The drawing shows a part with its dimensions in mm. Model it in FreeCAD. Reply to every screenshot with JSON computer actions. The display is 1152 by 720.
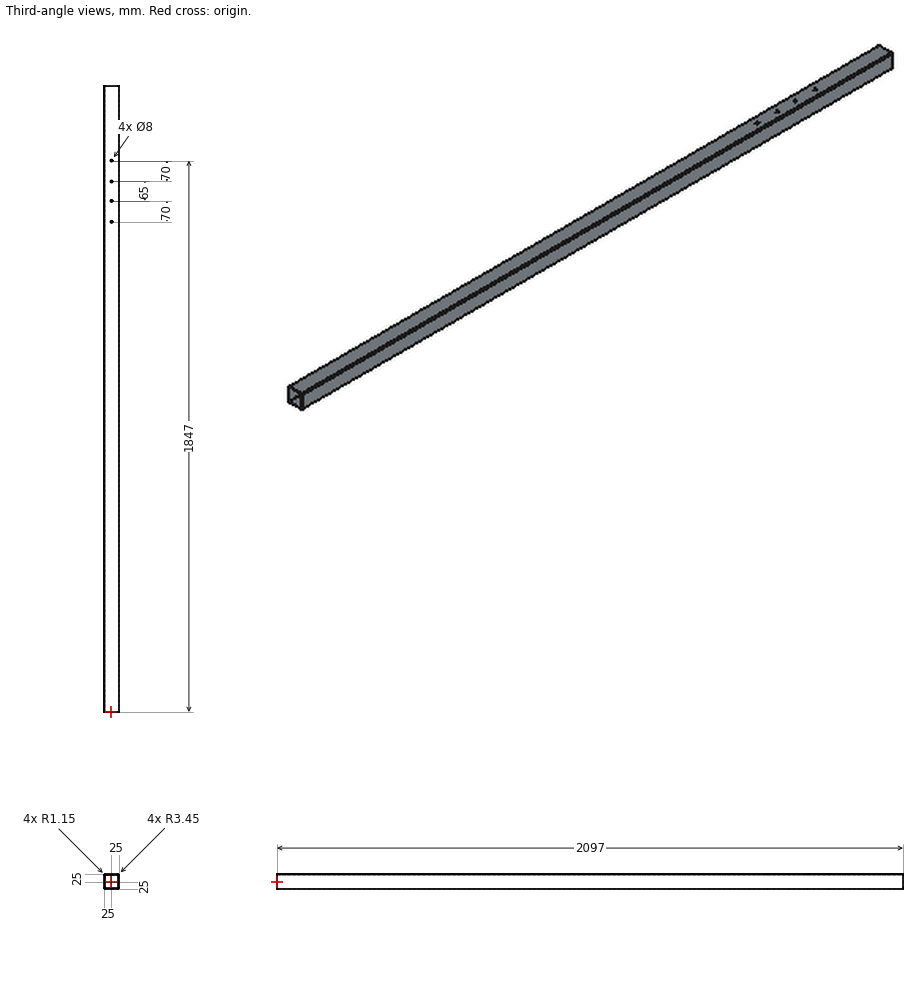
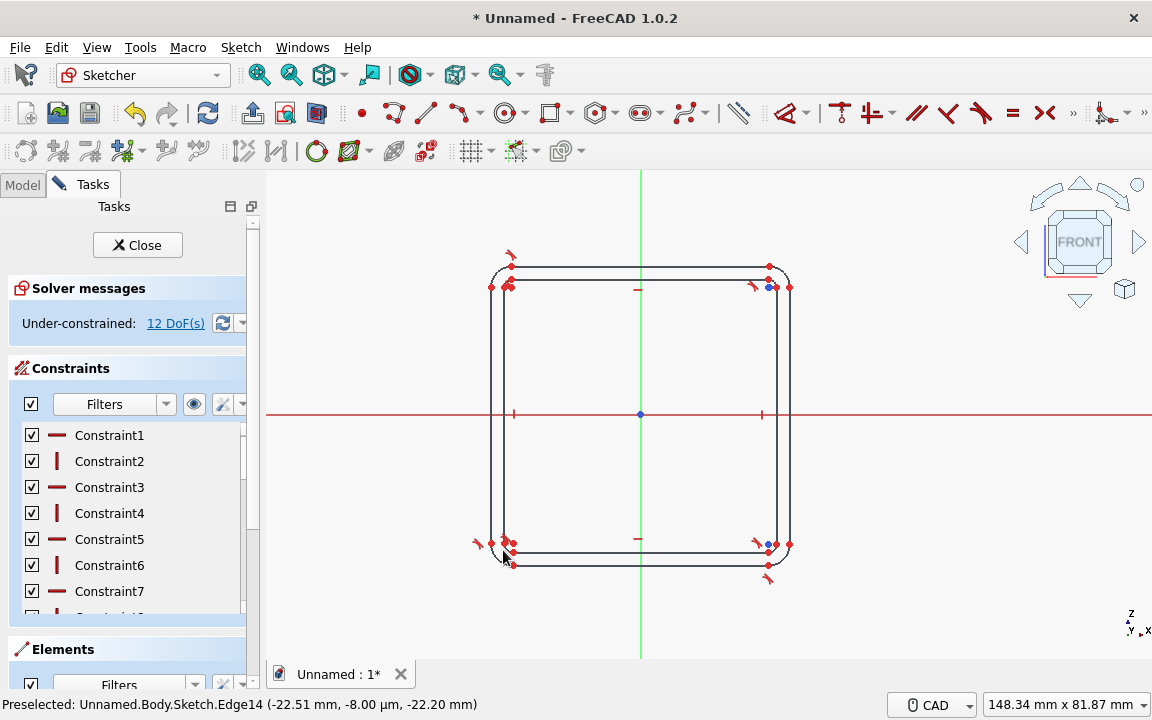
{"action": "scroll", "coordinate": [778, 563], "scroll_direction": "up", "scroll_amount": 2}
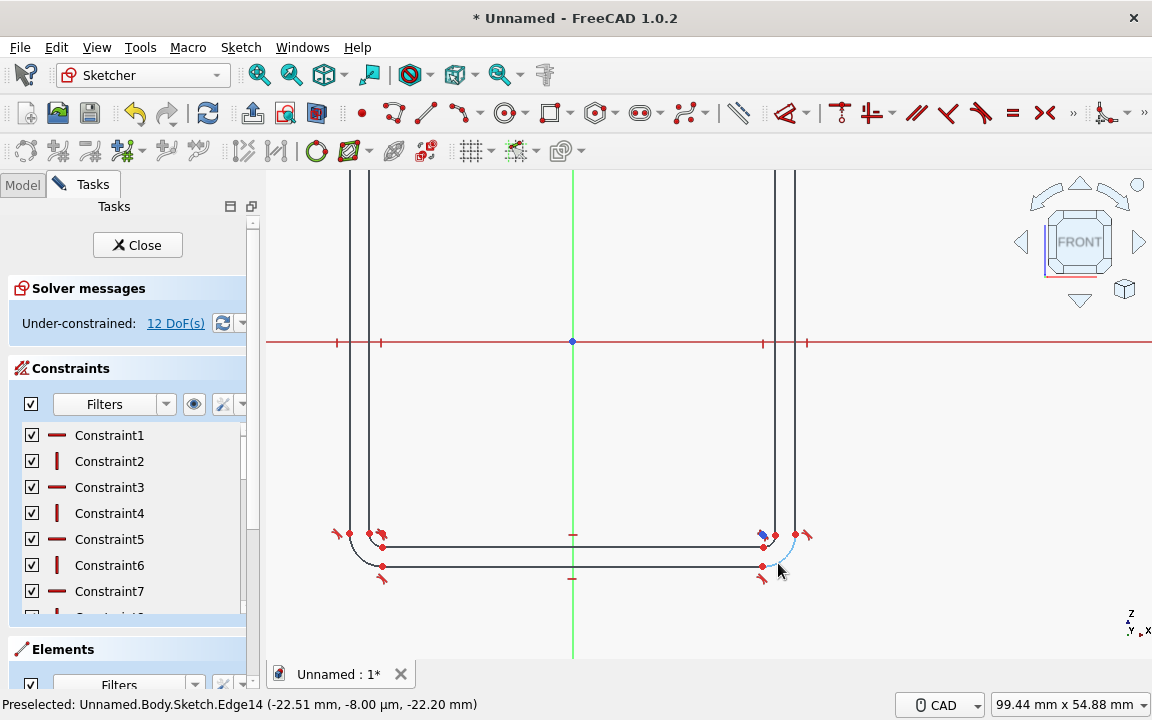
{"action": "left_click", "coordinate": [778, 563]}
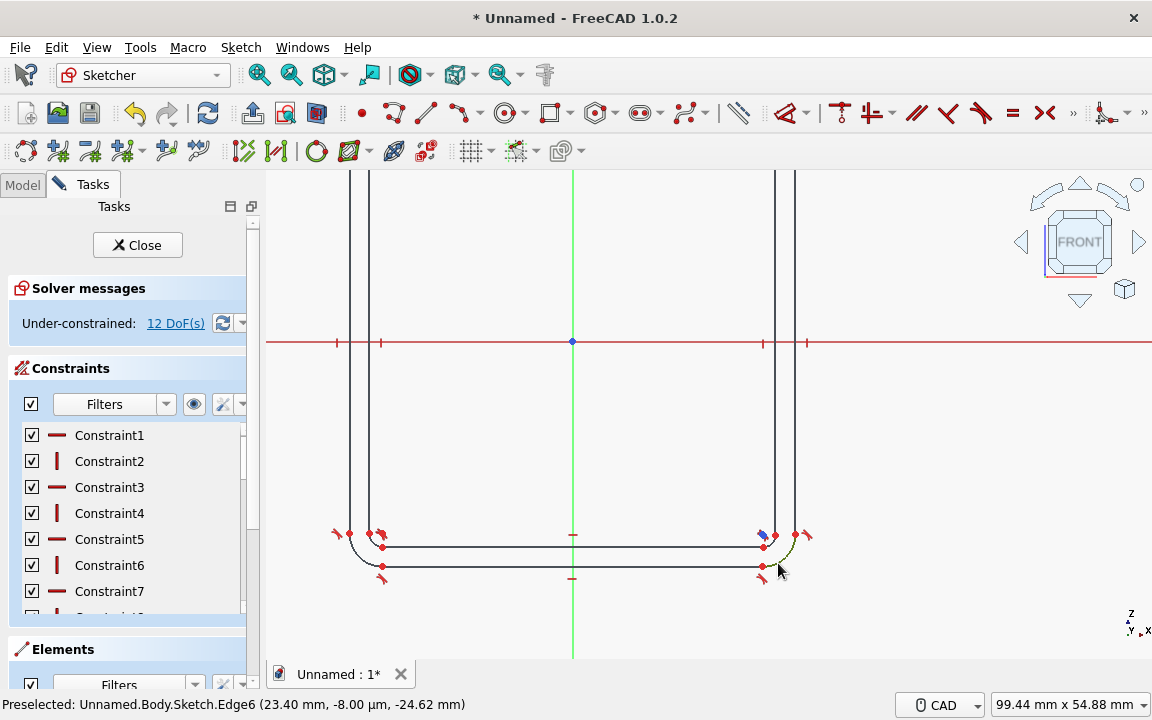
{"action": "scroll", "coordinate": [772, 544], "scroll_direction": "up", "scroll_amount": 3}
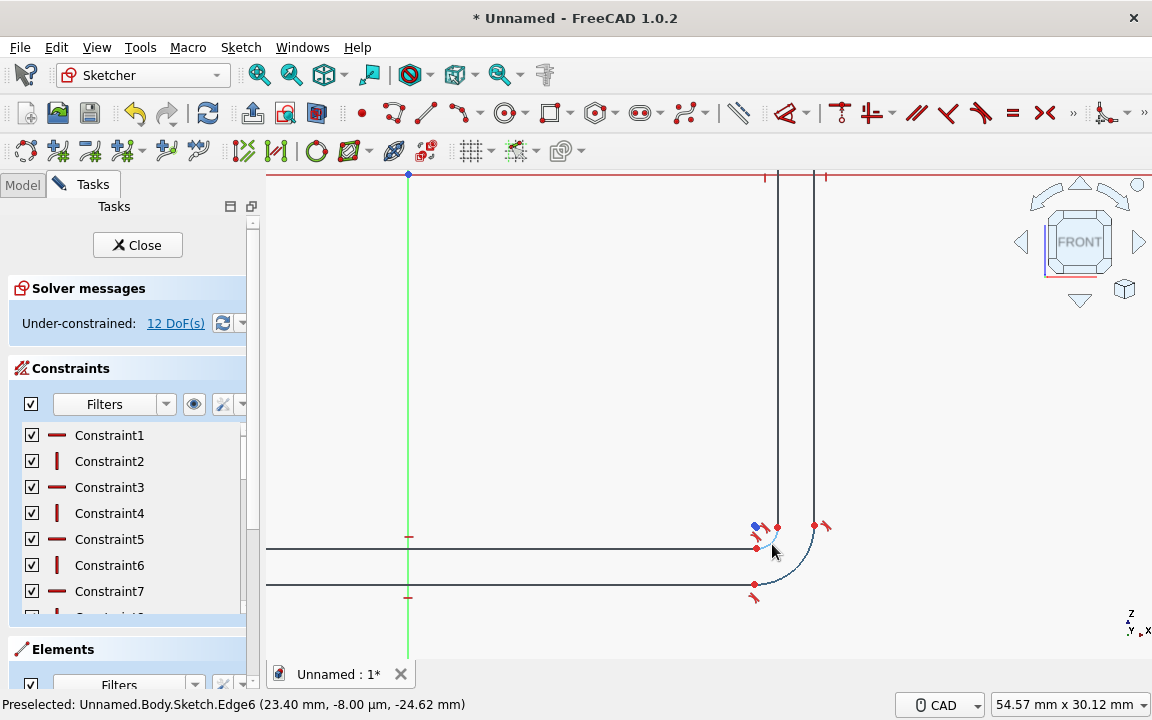
{"action": "left_click", "coordinate": [772, 543]}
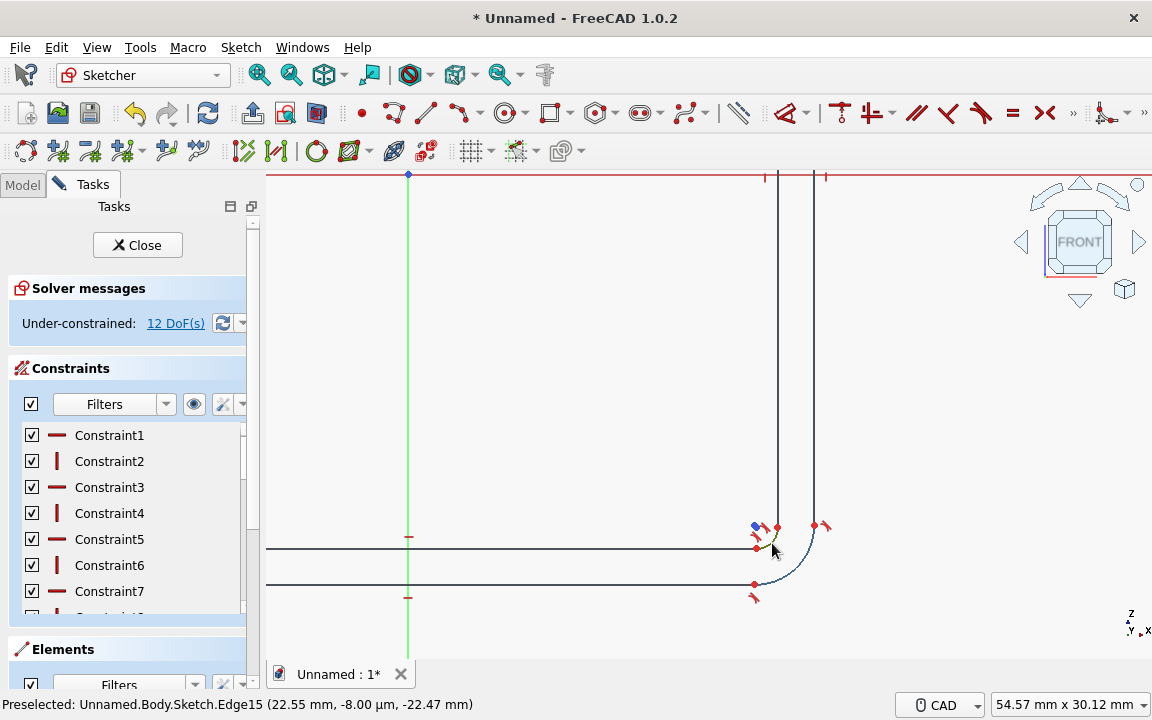
{"action": "left_click", "coordinate": [840, 114]}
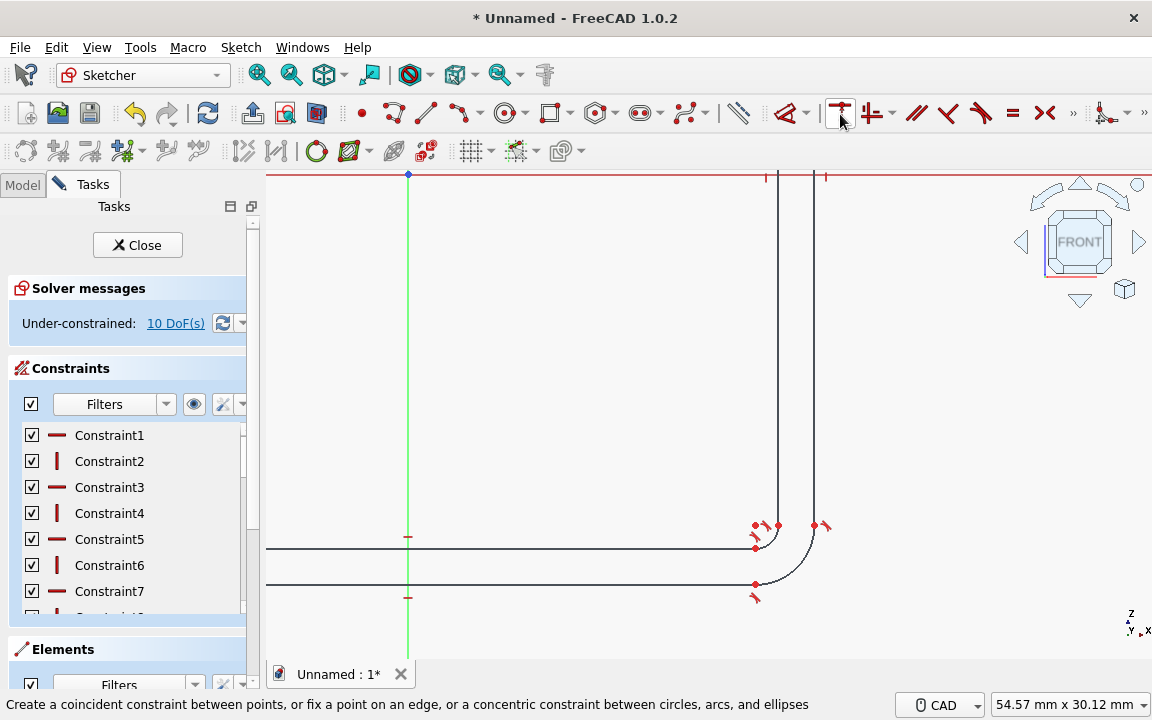
{"action": "scroll", "coordinate": [776, 554], "scroll_direction": "down", "scroll_amount": 5}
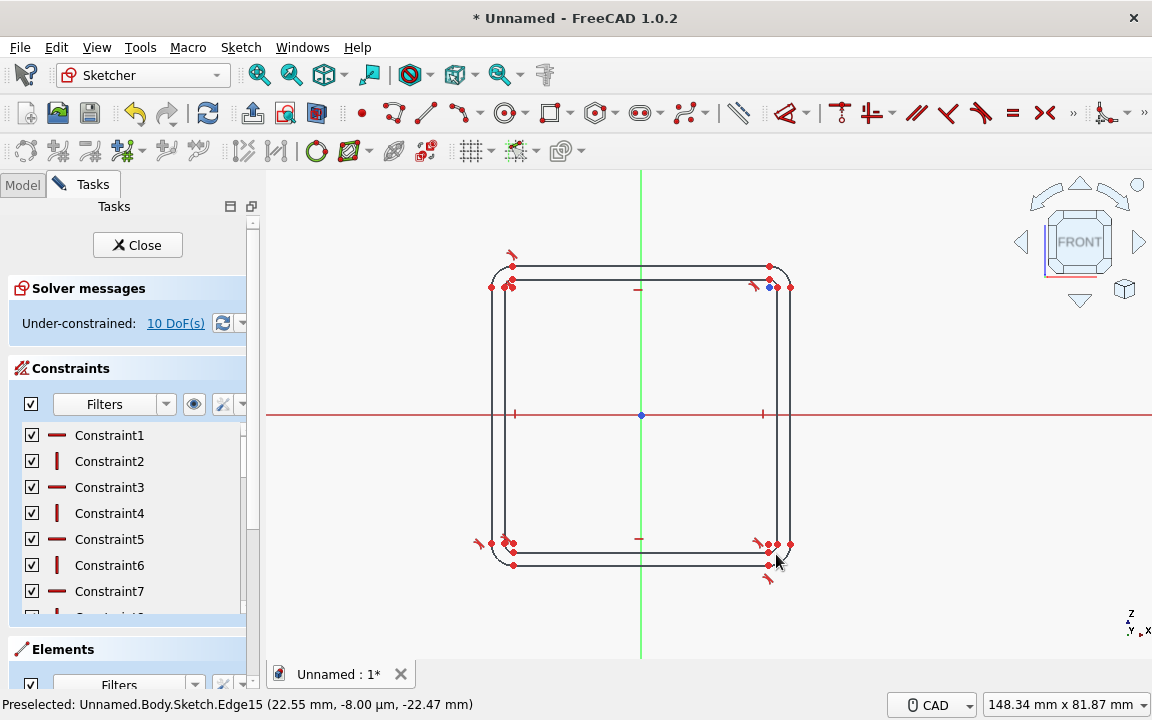
{"action": "scroll", "coordinate": [788, 278], "scroll_direction": "up", "scroll_amount": 2}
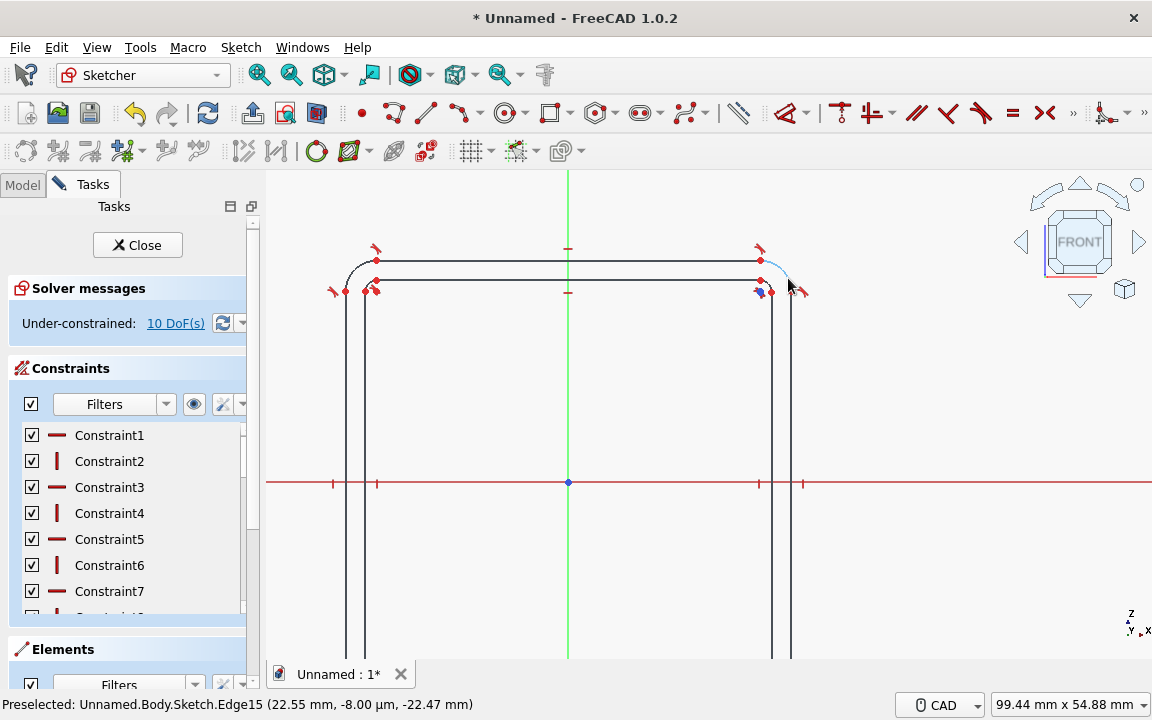
{"action": "left_click", "coordinate": [788, 278]}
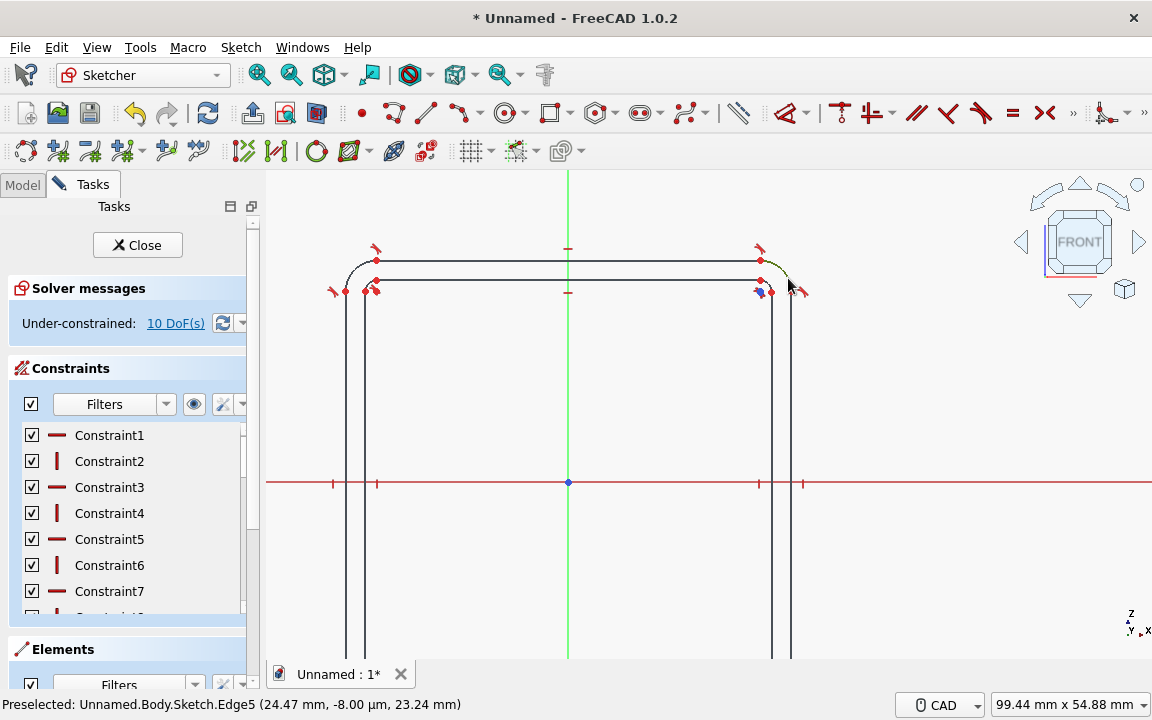
{"action": "scroll", "coordinate": [787, 277], "scroll_direction": "down", "scroll_amount": 2}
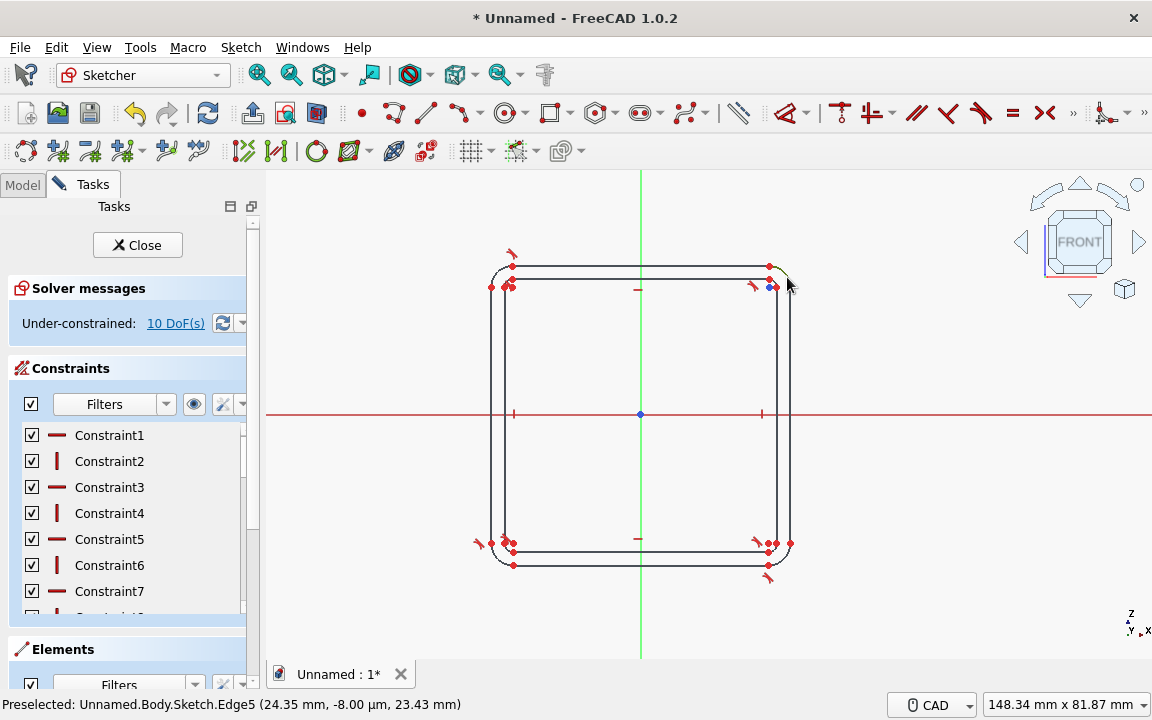
{"action": "scroll", "coordinate": [778, 563], "scroll_direction": "up", "scroll_amount": 2}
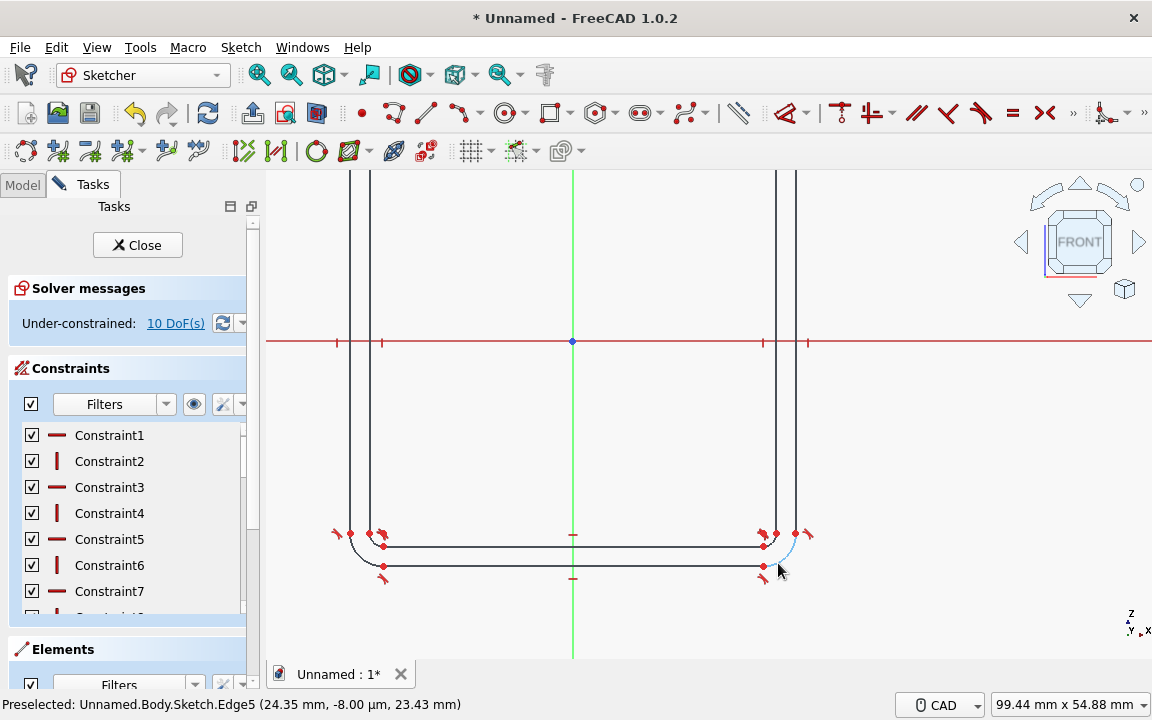
{"action": "left_click", "coordinate": [778, 563]}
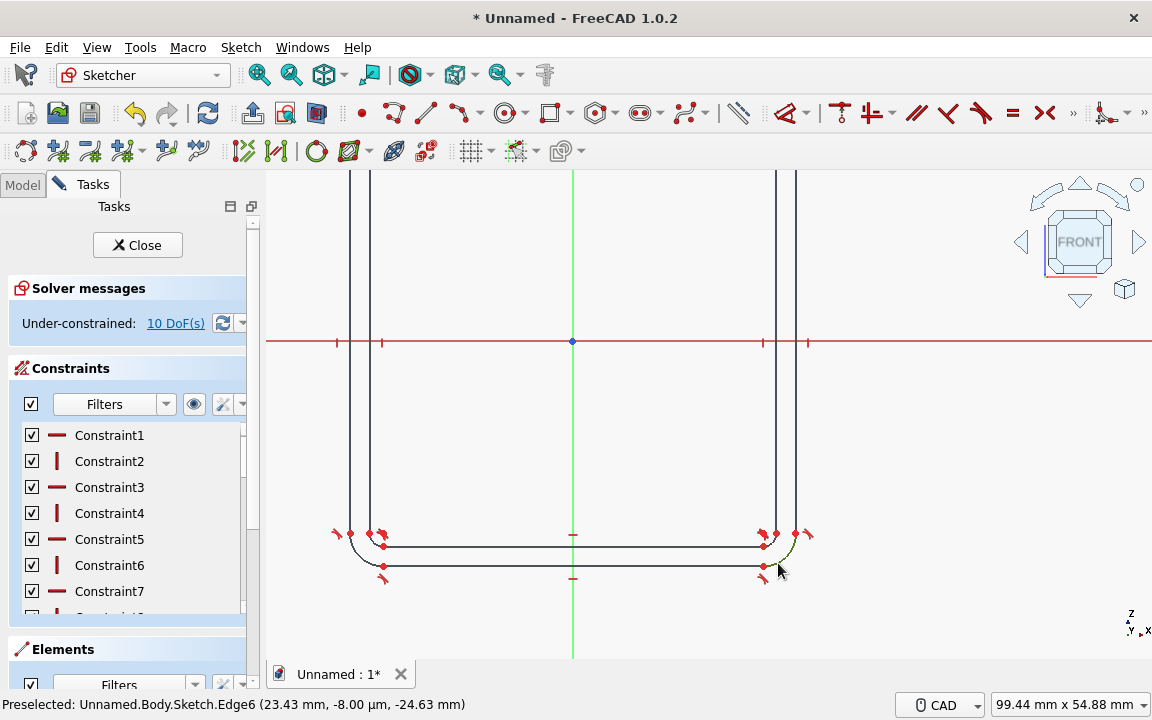
{"action": "left_click", "coordinate": [354, 548]}